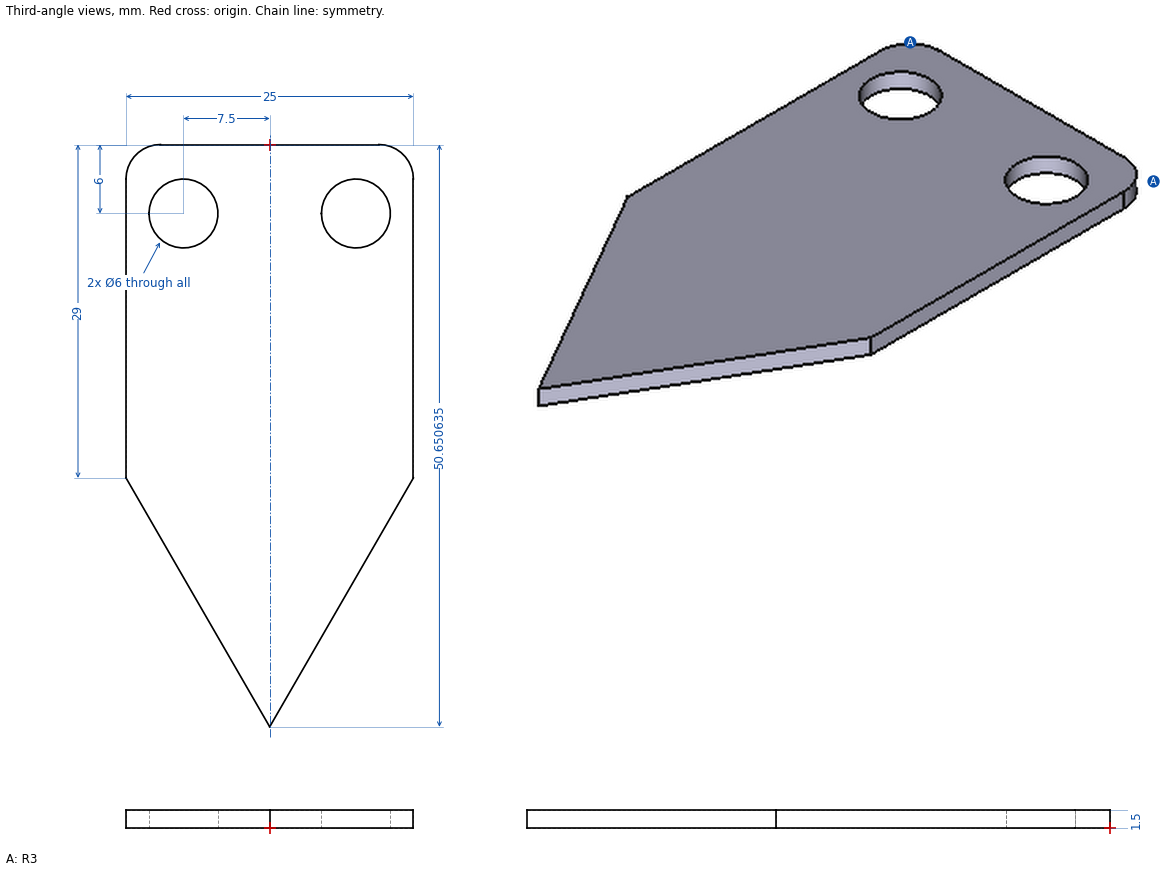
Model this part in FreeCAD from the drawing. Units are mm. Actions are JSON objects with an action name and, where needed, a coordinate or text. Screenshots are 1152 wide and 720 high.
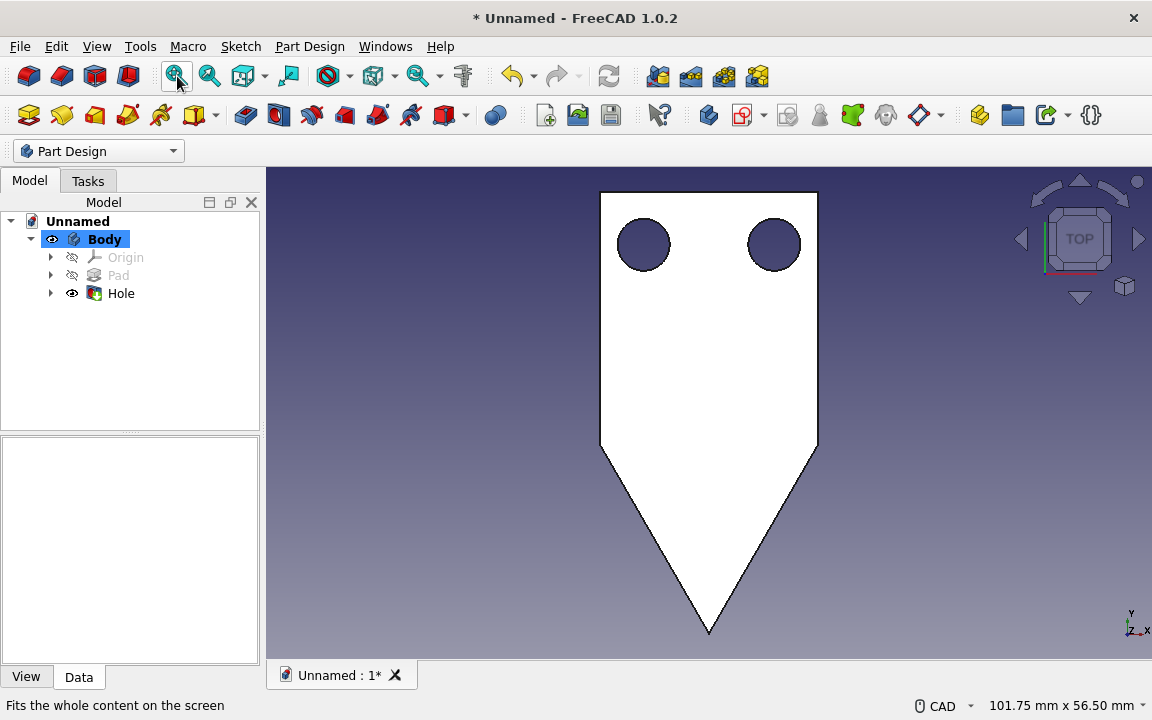
{"action": "key", "text": "1"}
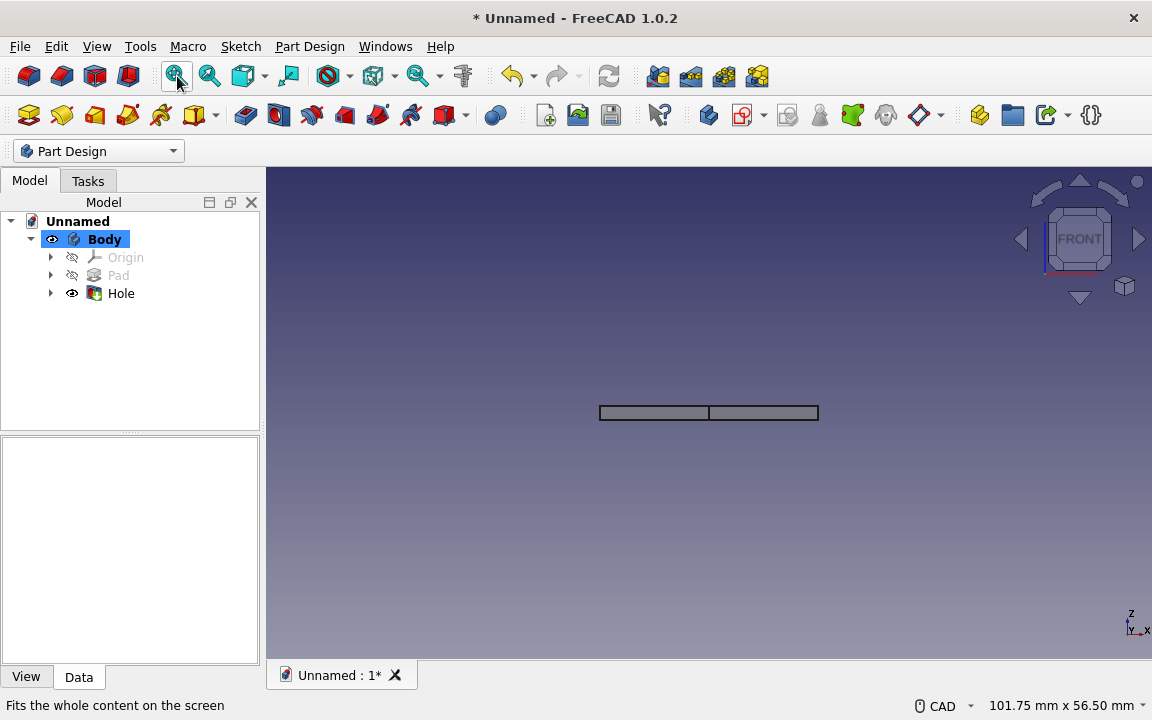
{"action": "left_click", "coordinate": [177, 76]}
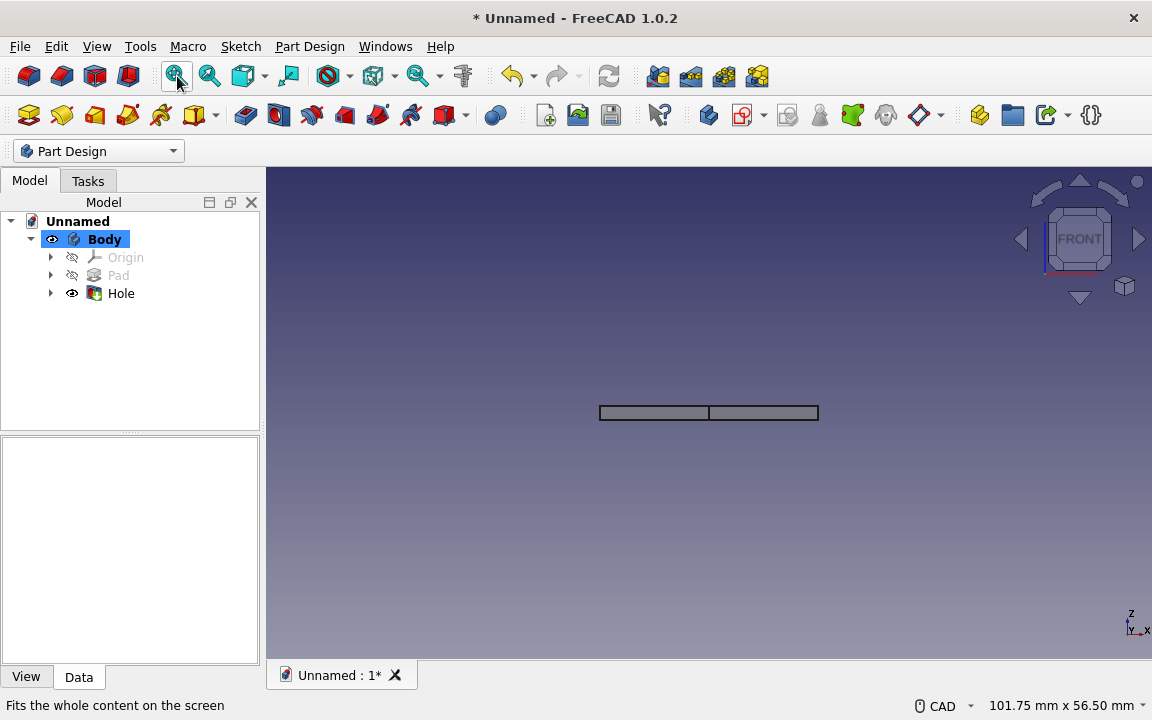
{"action": "scroll", "coordinate": [600, 412], "scroll_direction": "up", "scroll_amount": 6}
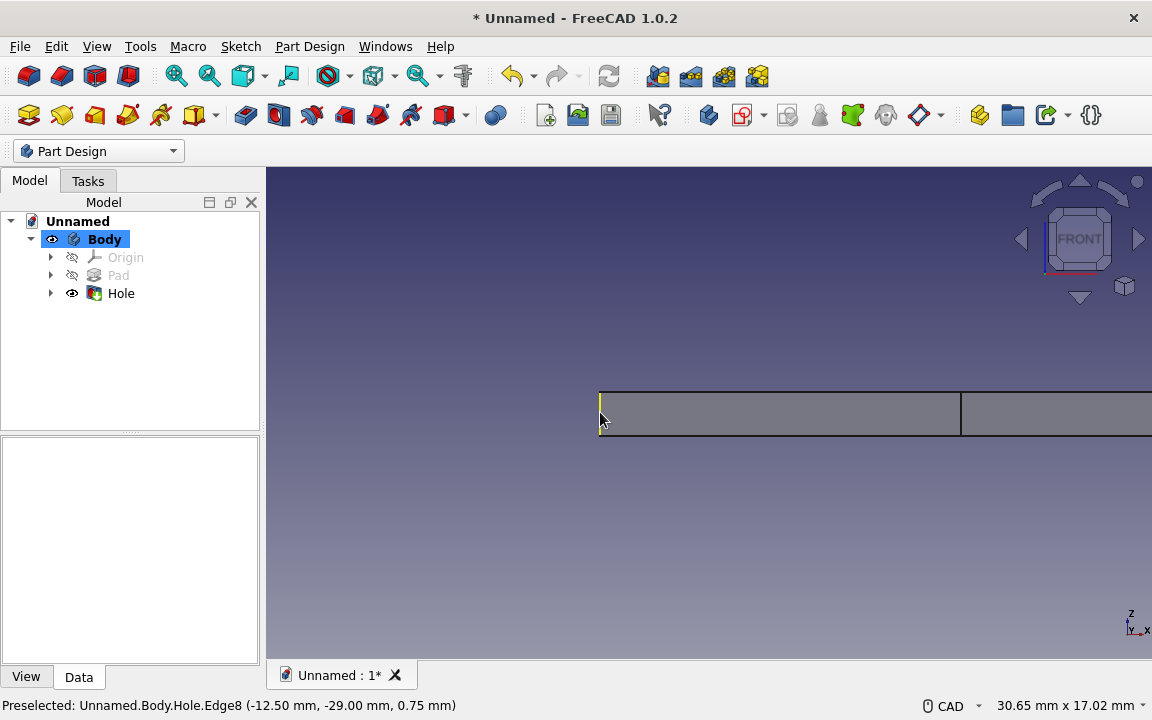
{"action": "left_click", "coordinate": [177, 76]}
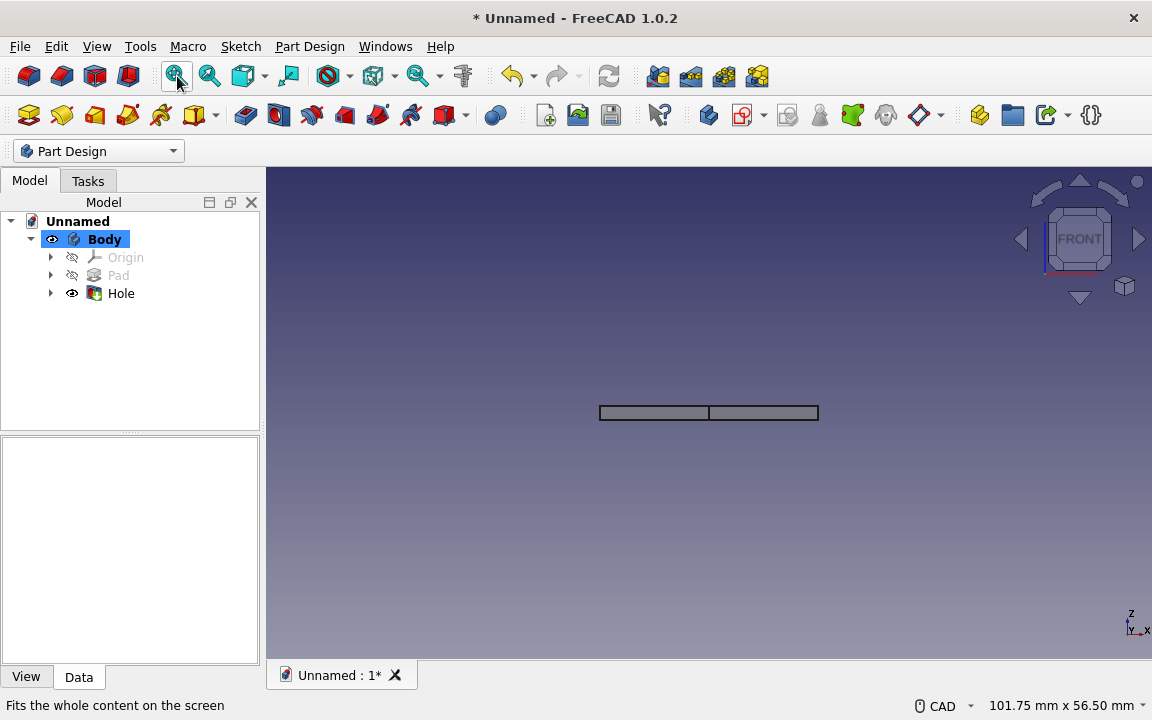
{"action": "key", "text": "3"}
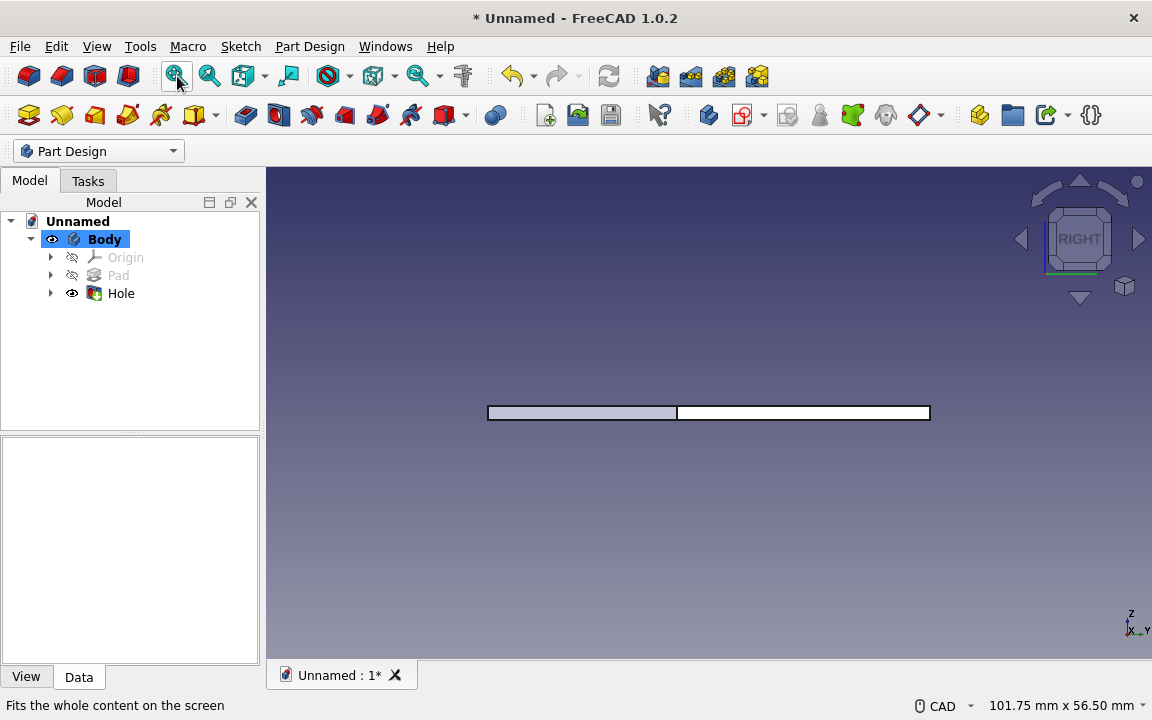
{"action": "left_click", "coordinate": [930, 412]}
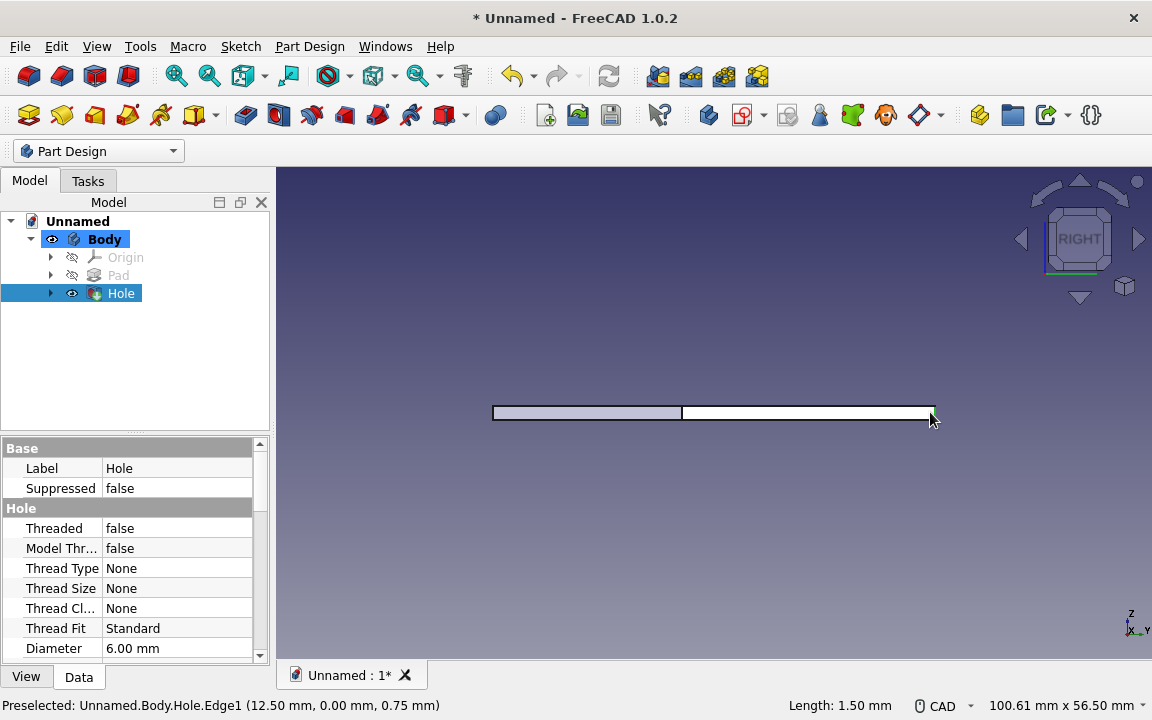
{"action": "scroll", "coordinate": [935, 412], "scroll_direction": "up", "scroll_amount": 6}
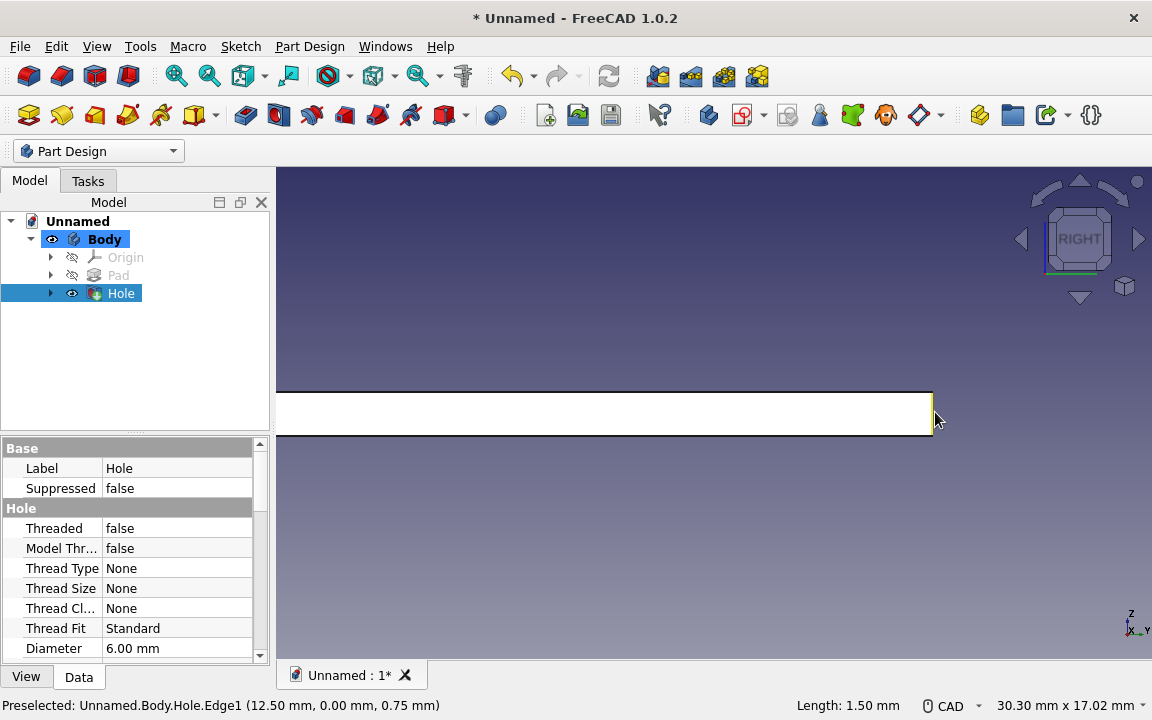
{"action": "left_click", "coordinate": [177, 76]}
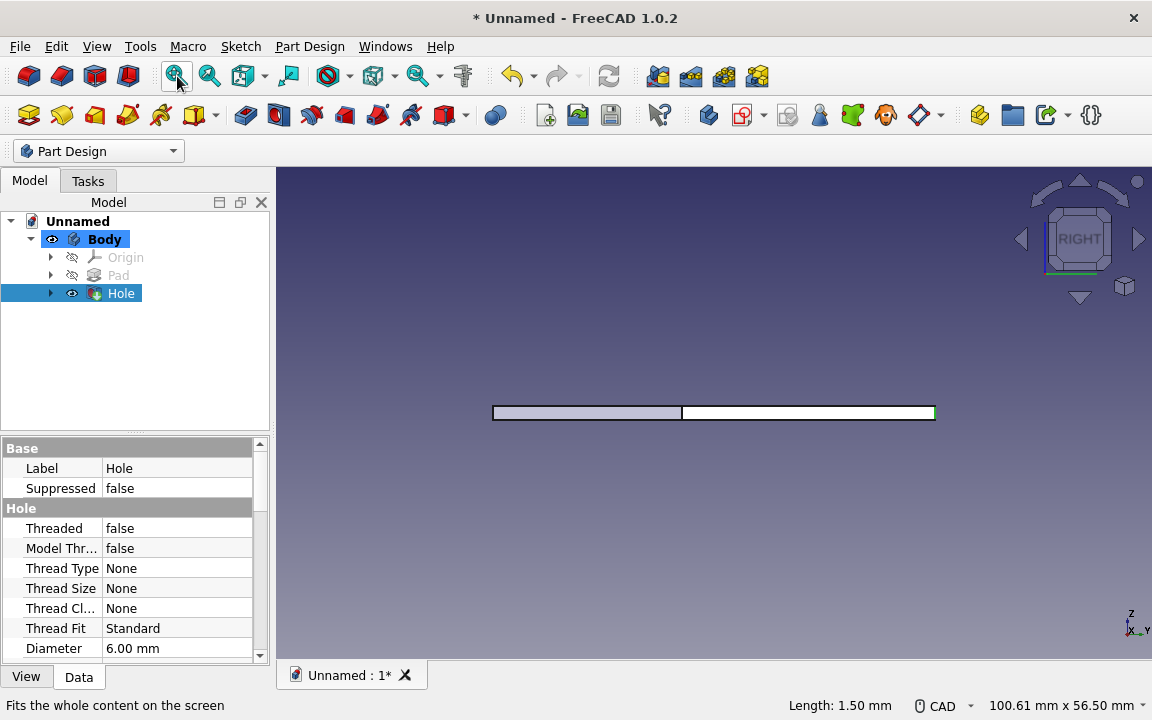
{"action": "key", "text": "5"}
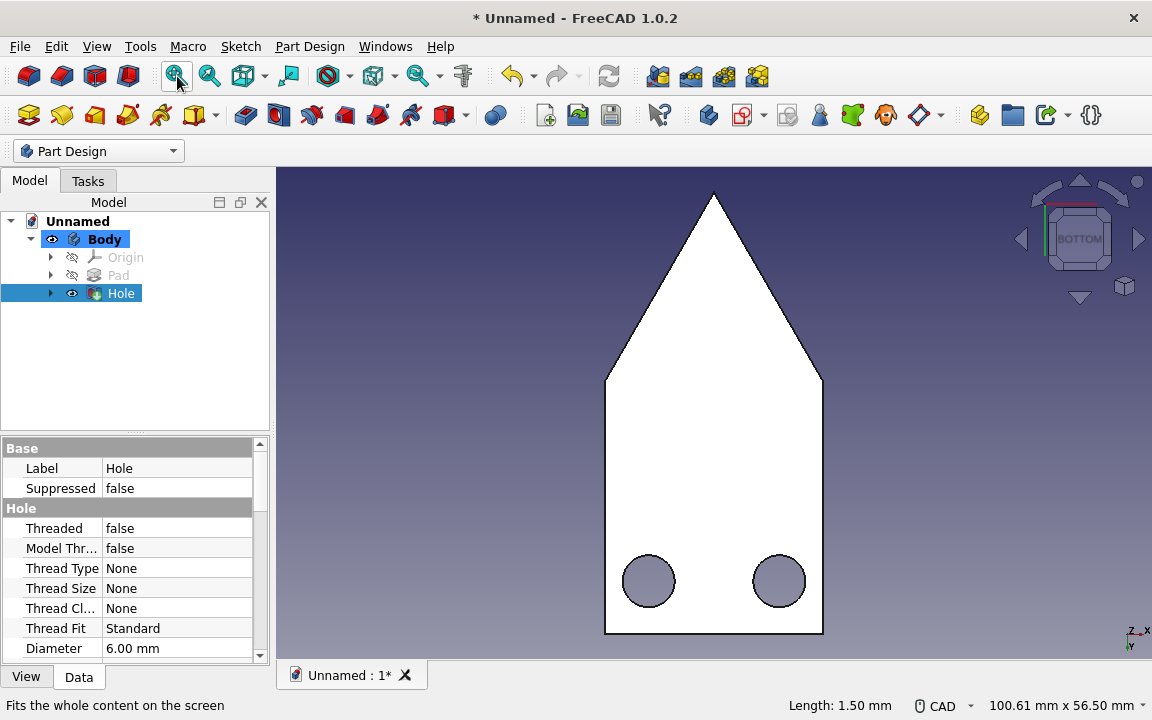
{"action": "key", "text": "4"}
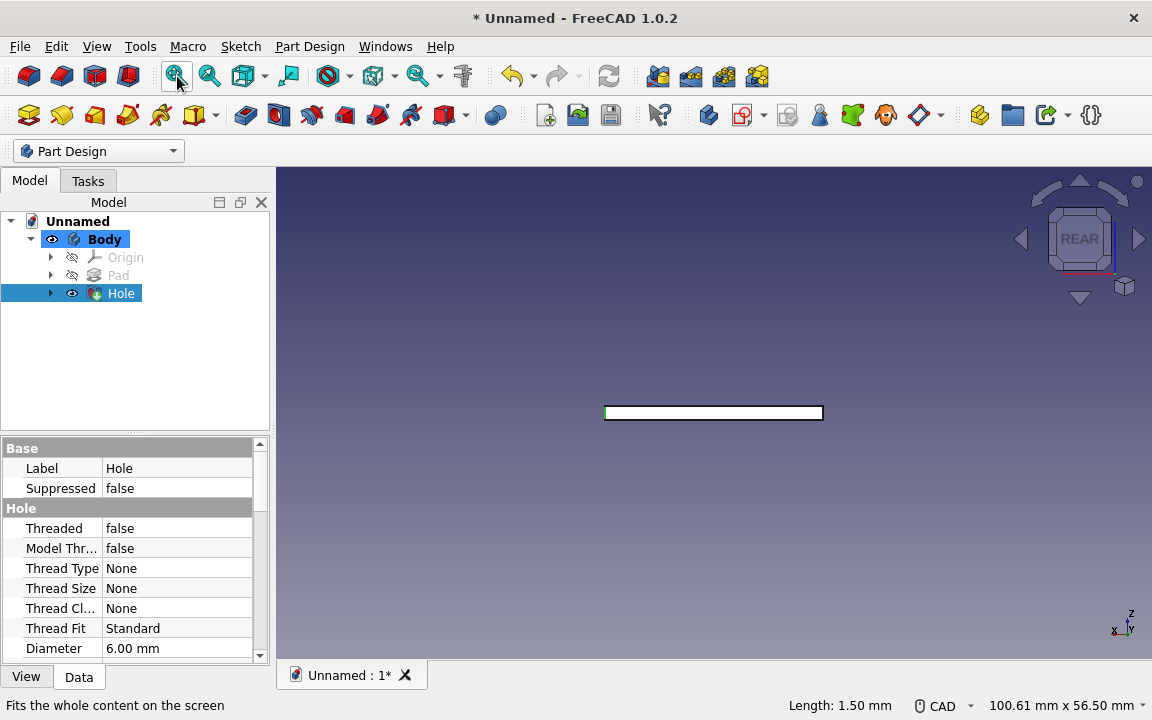
{"action": "left_click", "coordinate": [177, 76]}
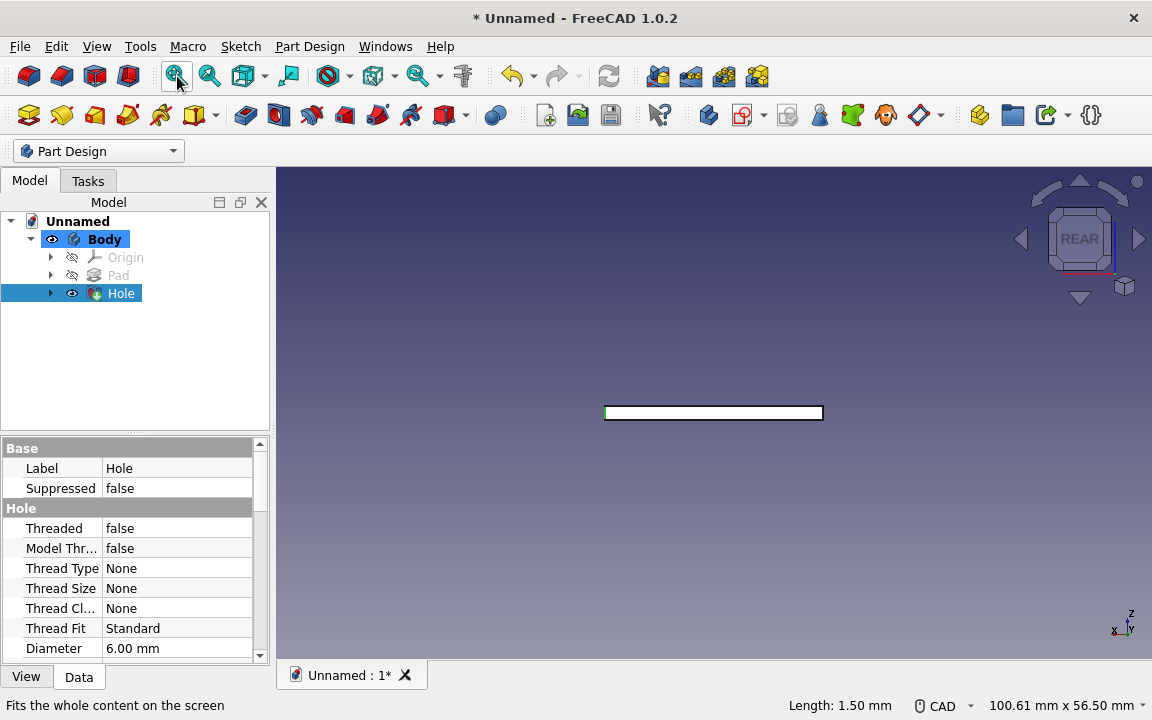
{"action": "left_click", "coordinate": [823, 412], "text": "ctrl"}